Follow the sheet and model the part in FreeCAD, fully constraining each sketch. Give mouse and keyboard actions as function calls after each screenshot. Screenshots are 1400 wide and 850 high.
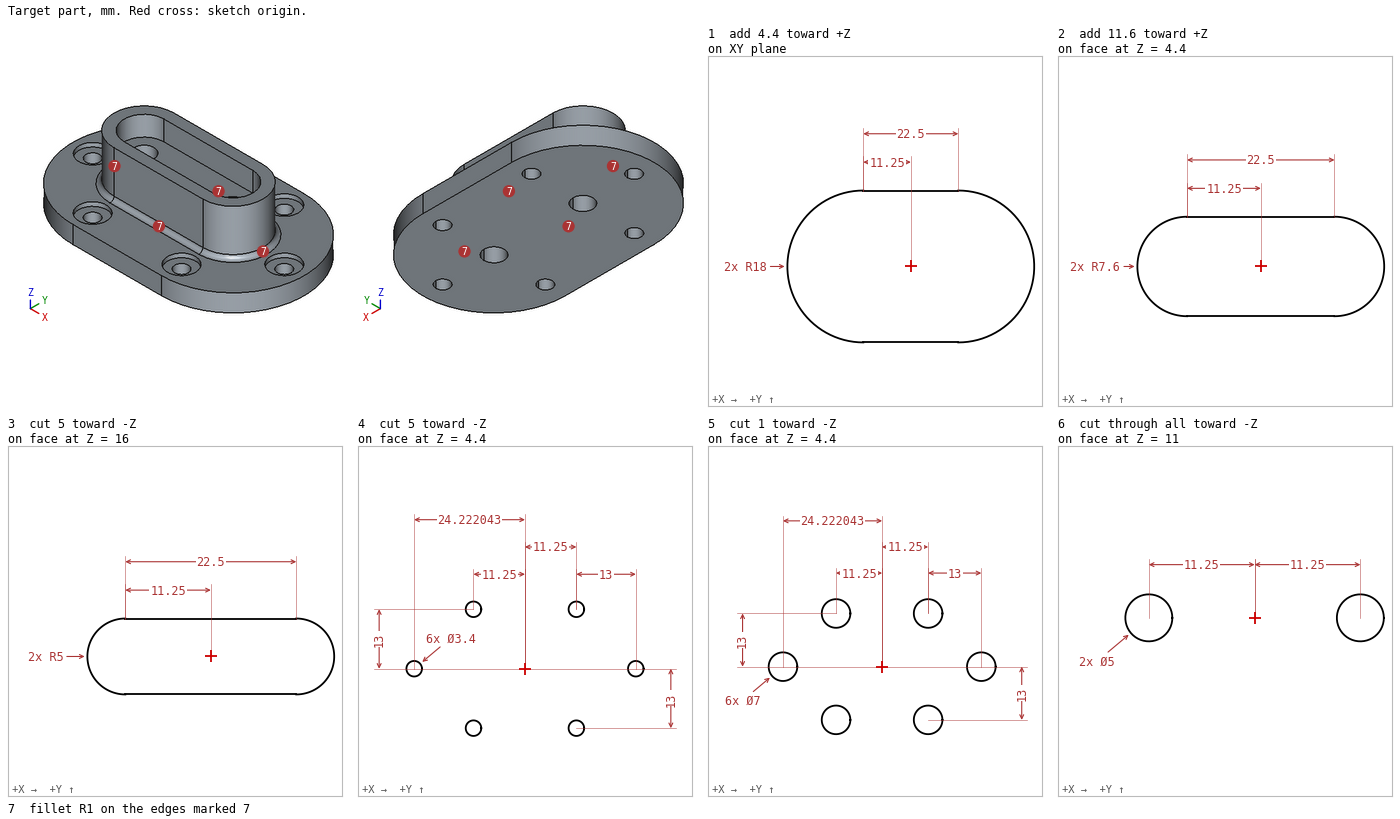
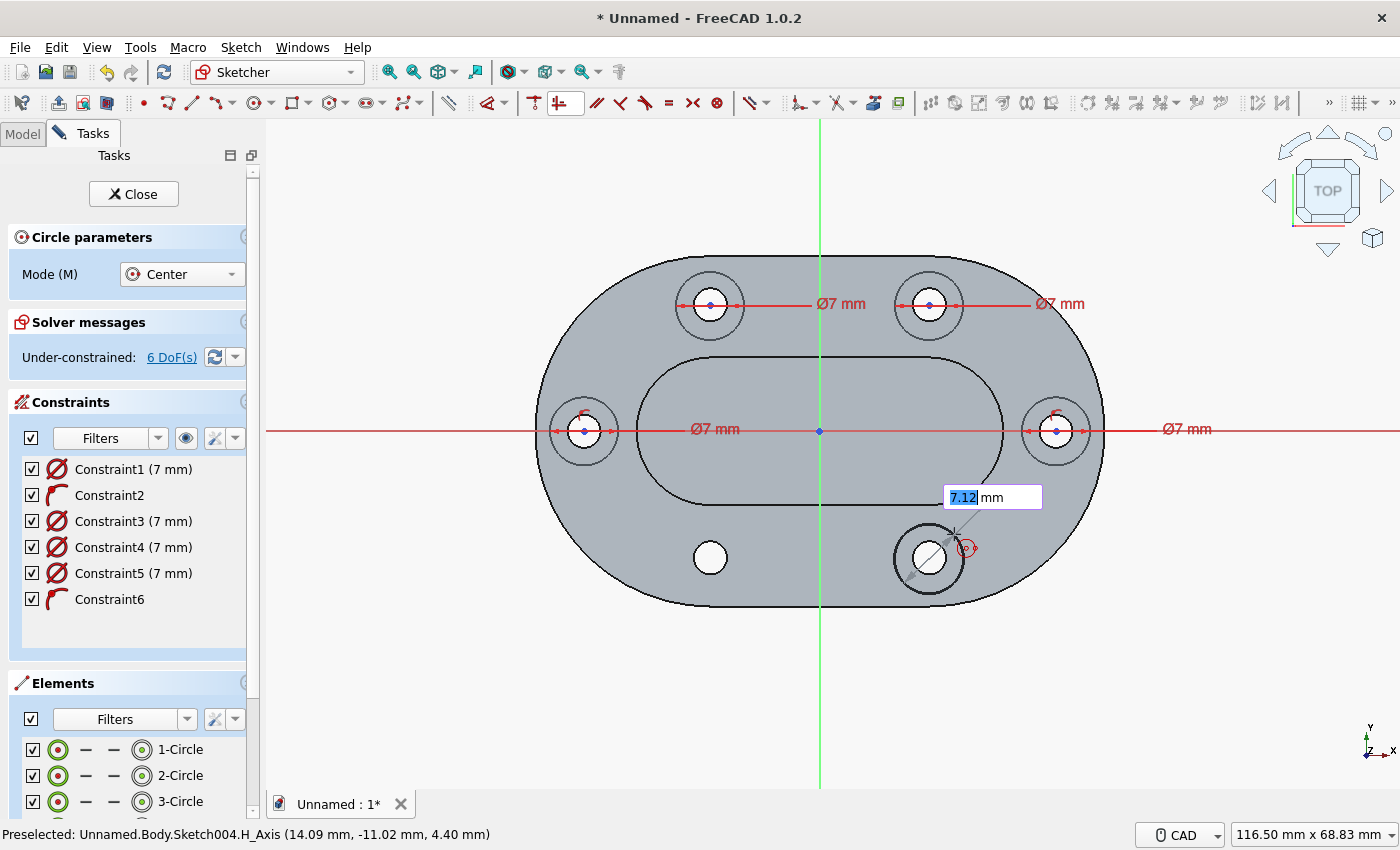
text(7)
key(Return)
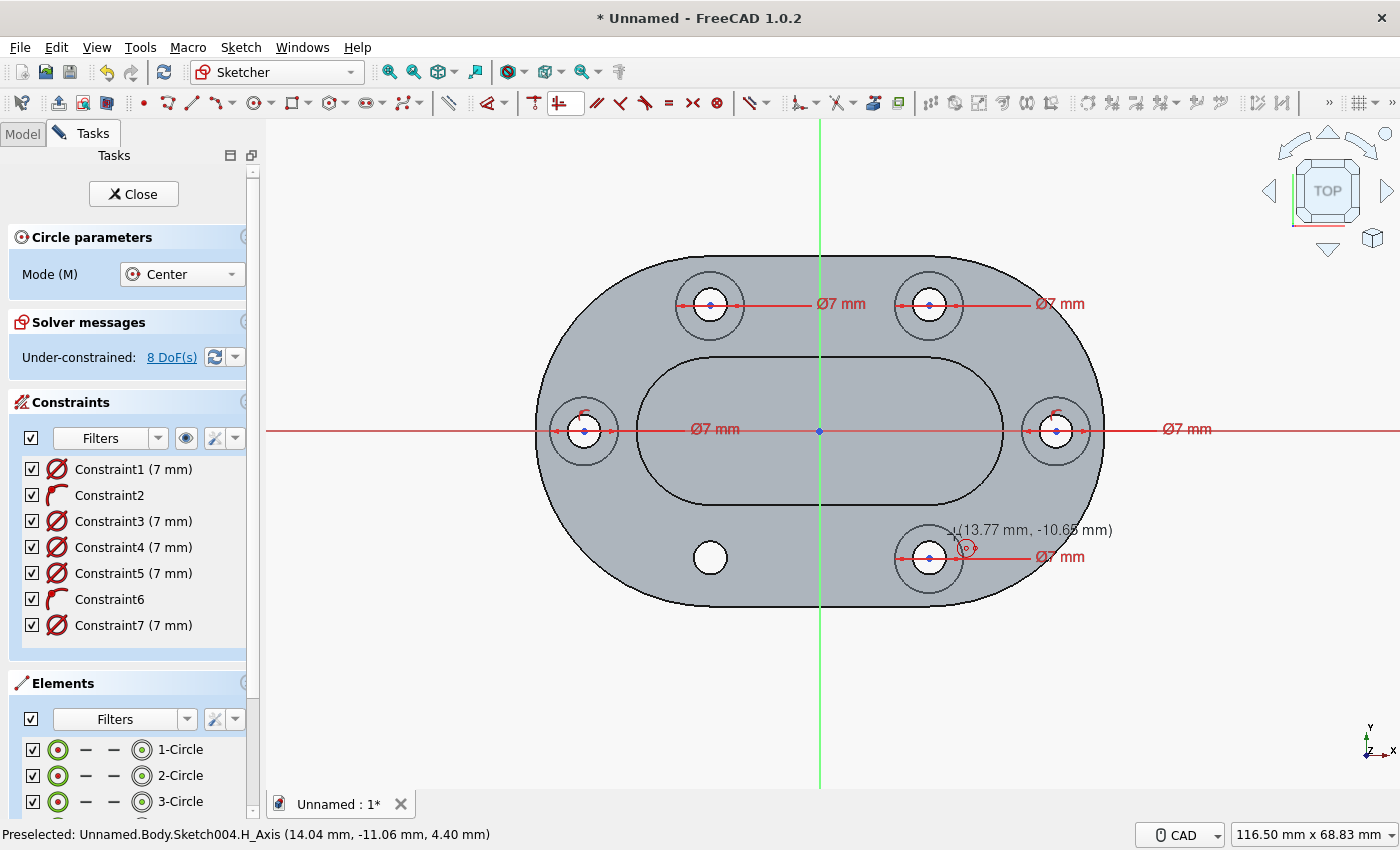
click(710, 558)
move(734, 534)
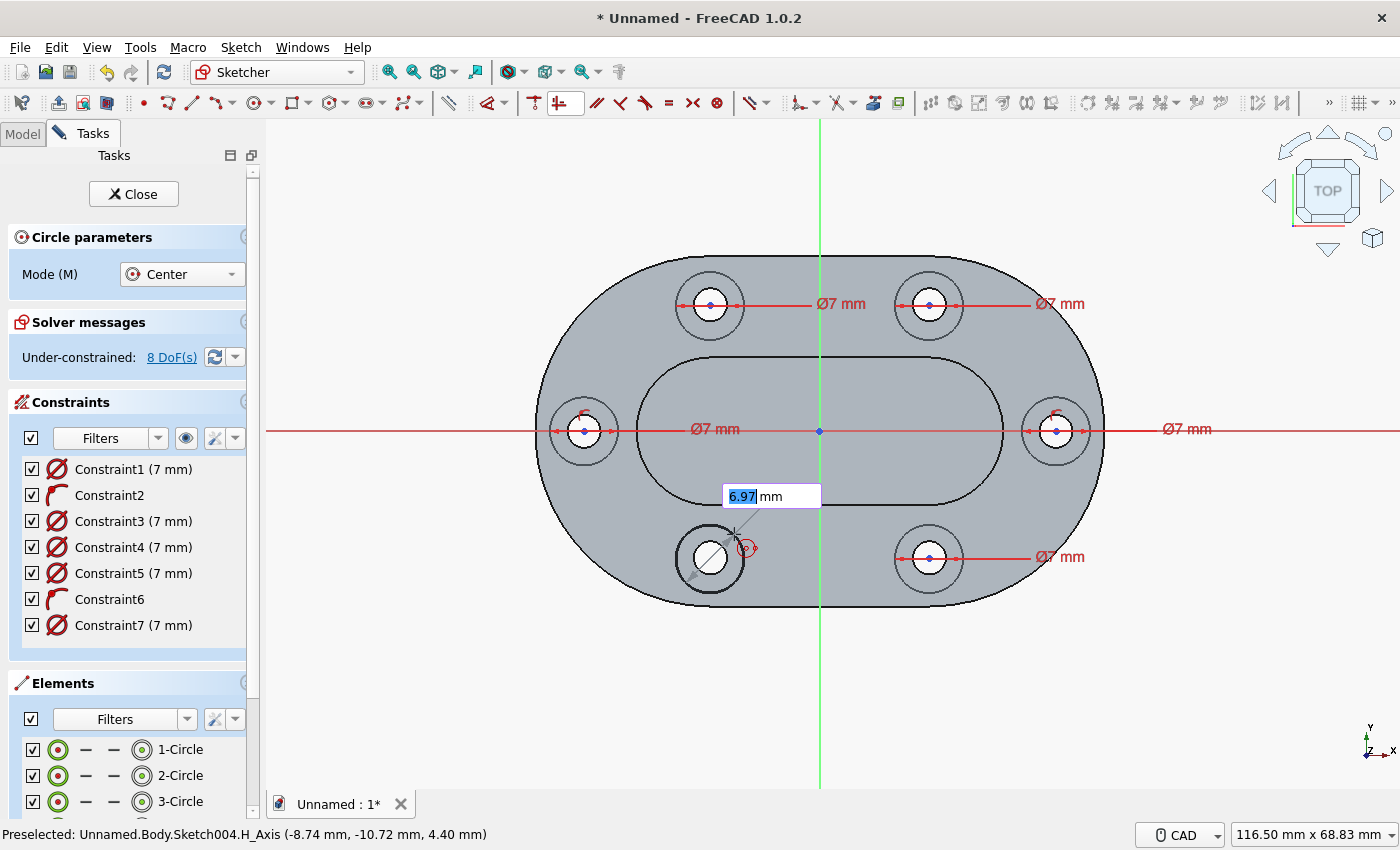
text(7)
key(Return)
key(Escape)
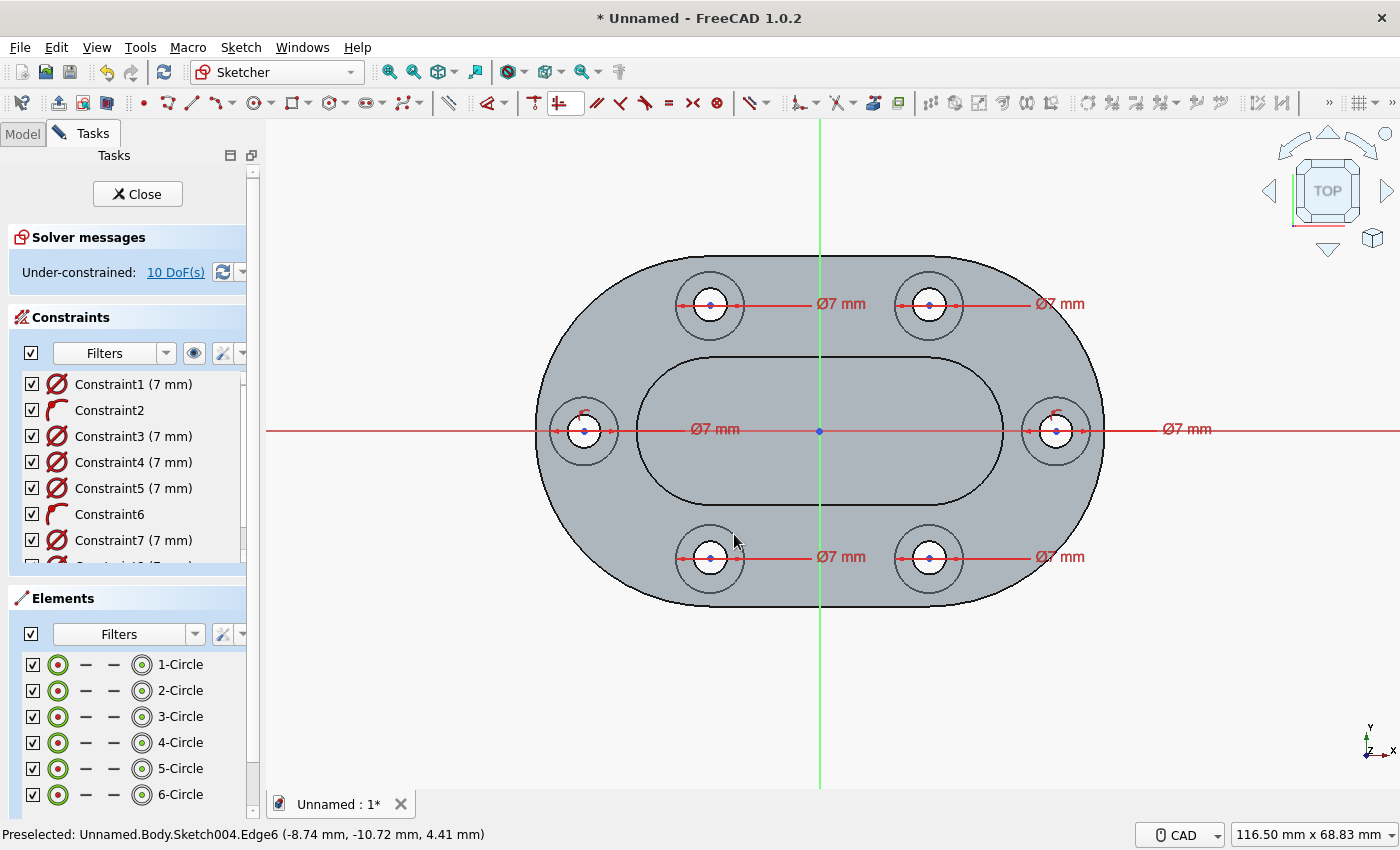
click(710, 306)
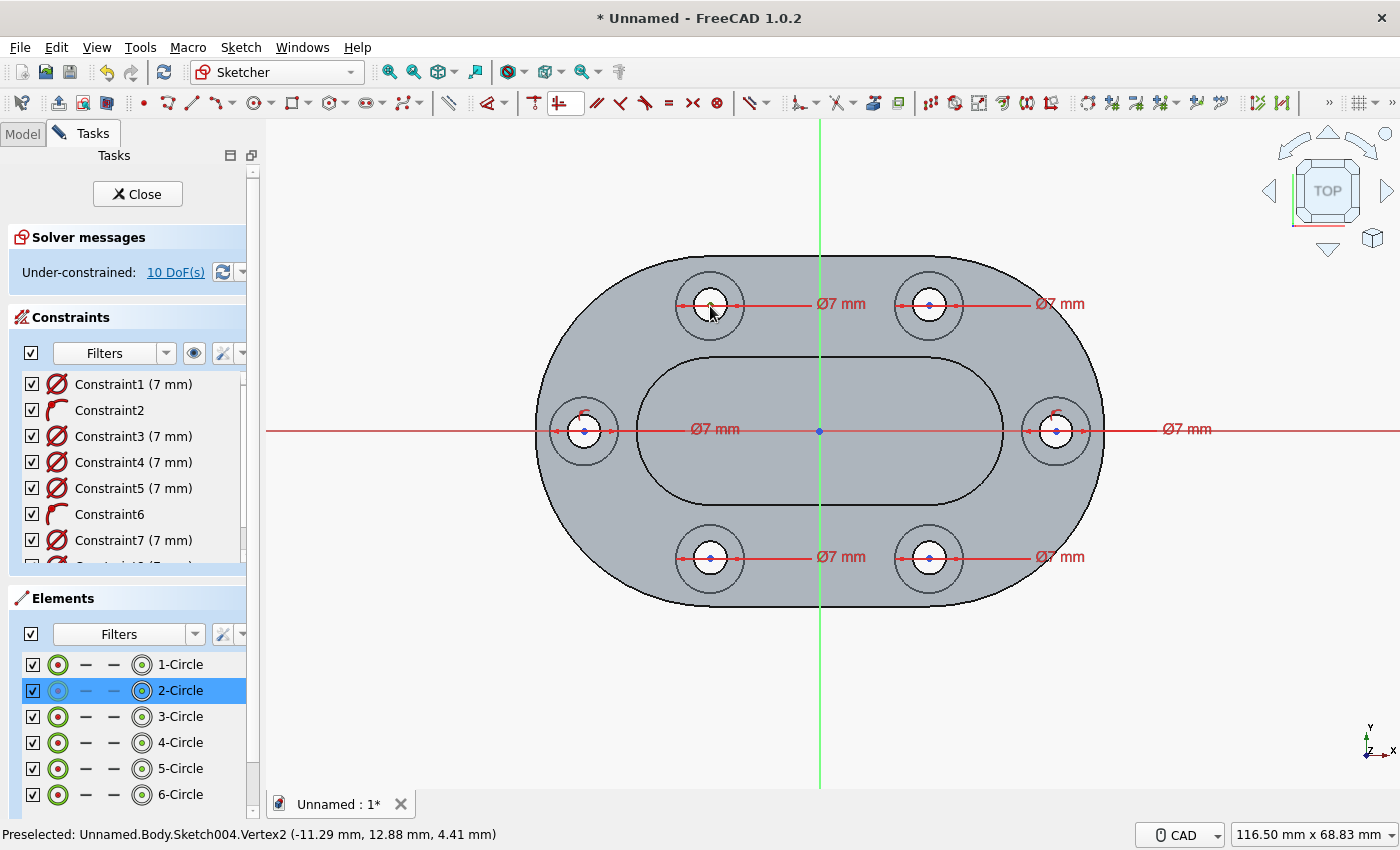
click(929, 306)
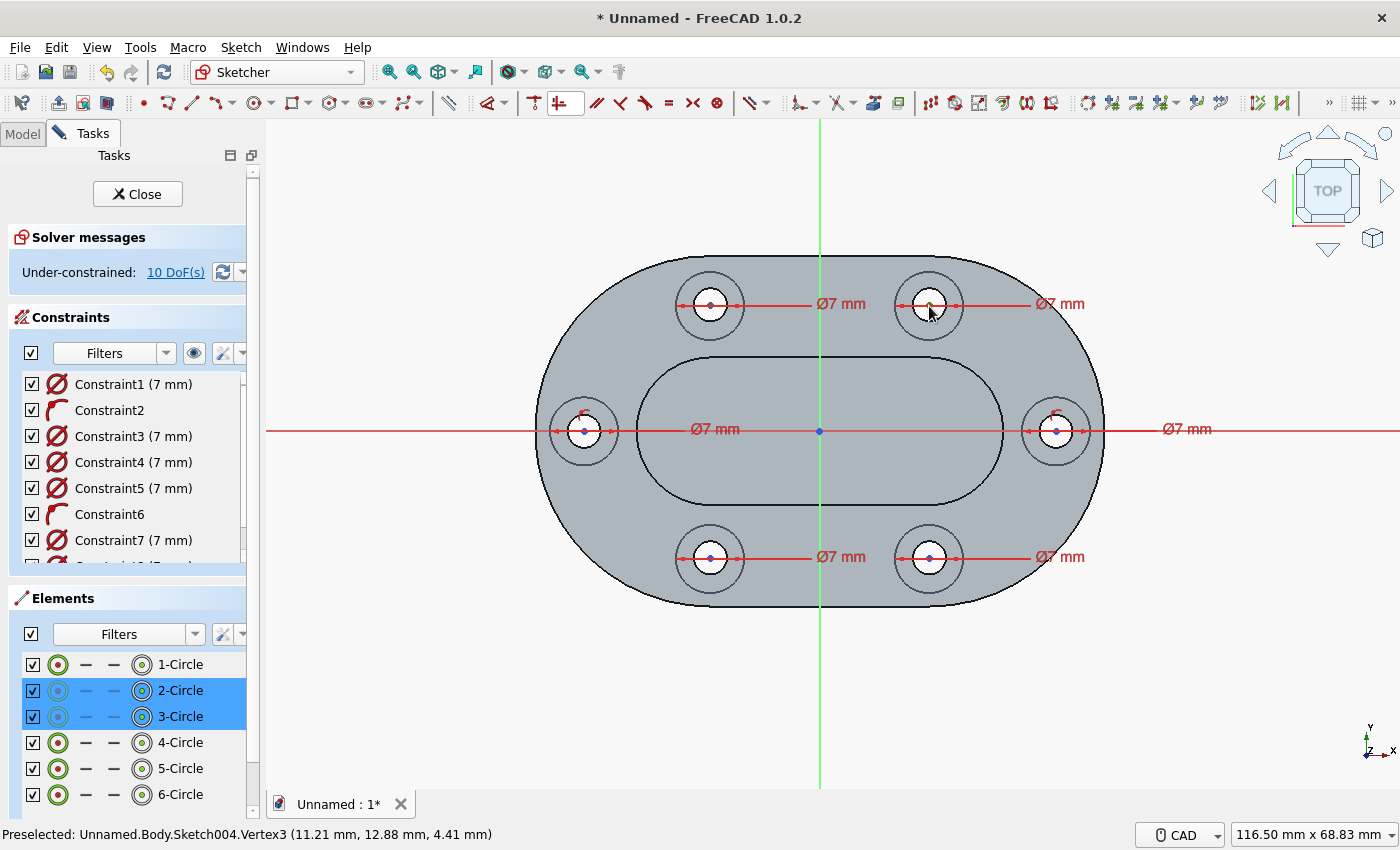
click(578, 104)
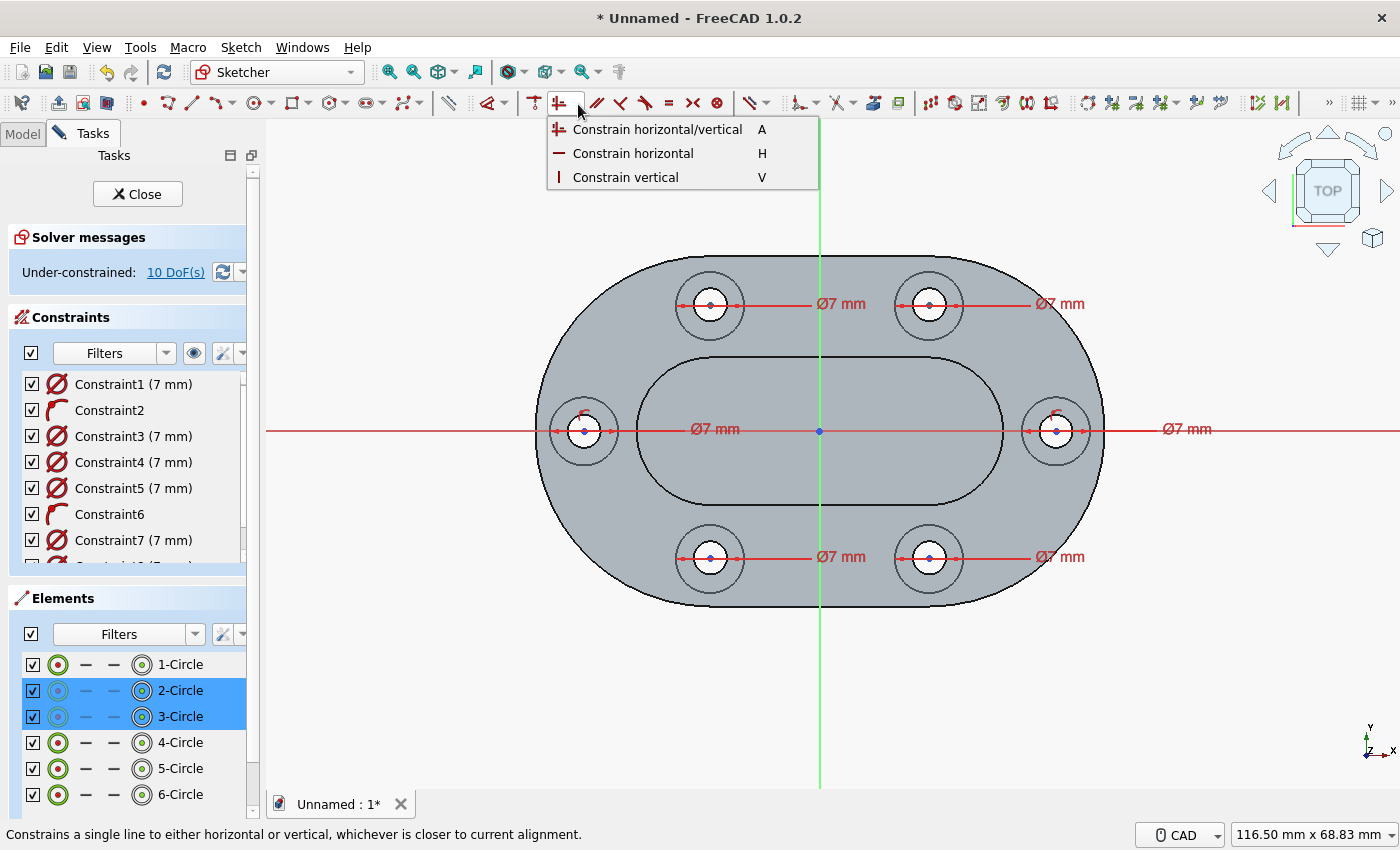
click(683, 153)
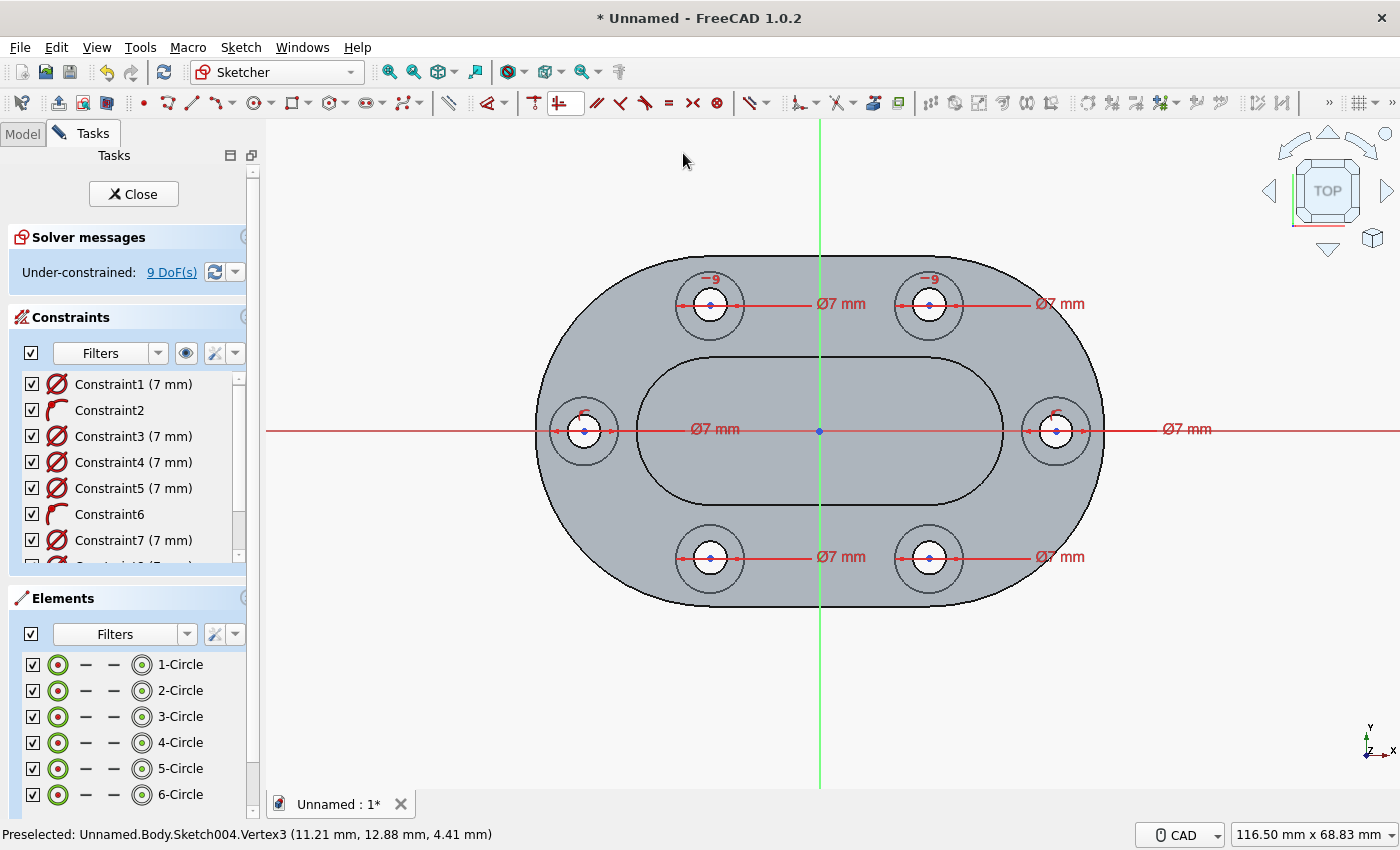
click(929, 306)